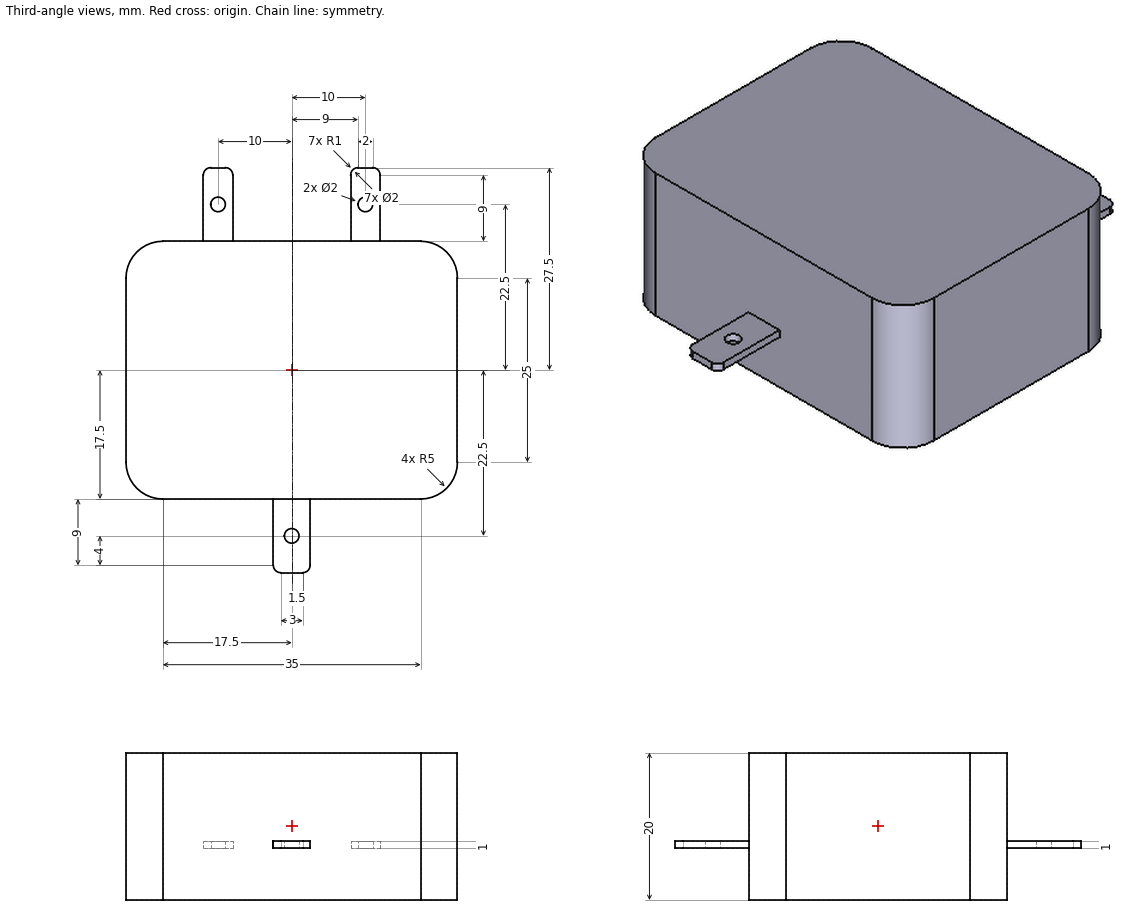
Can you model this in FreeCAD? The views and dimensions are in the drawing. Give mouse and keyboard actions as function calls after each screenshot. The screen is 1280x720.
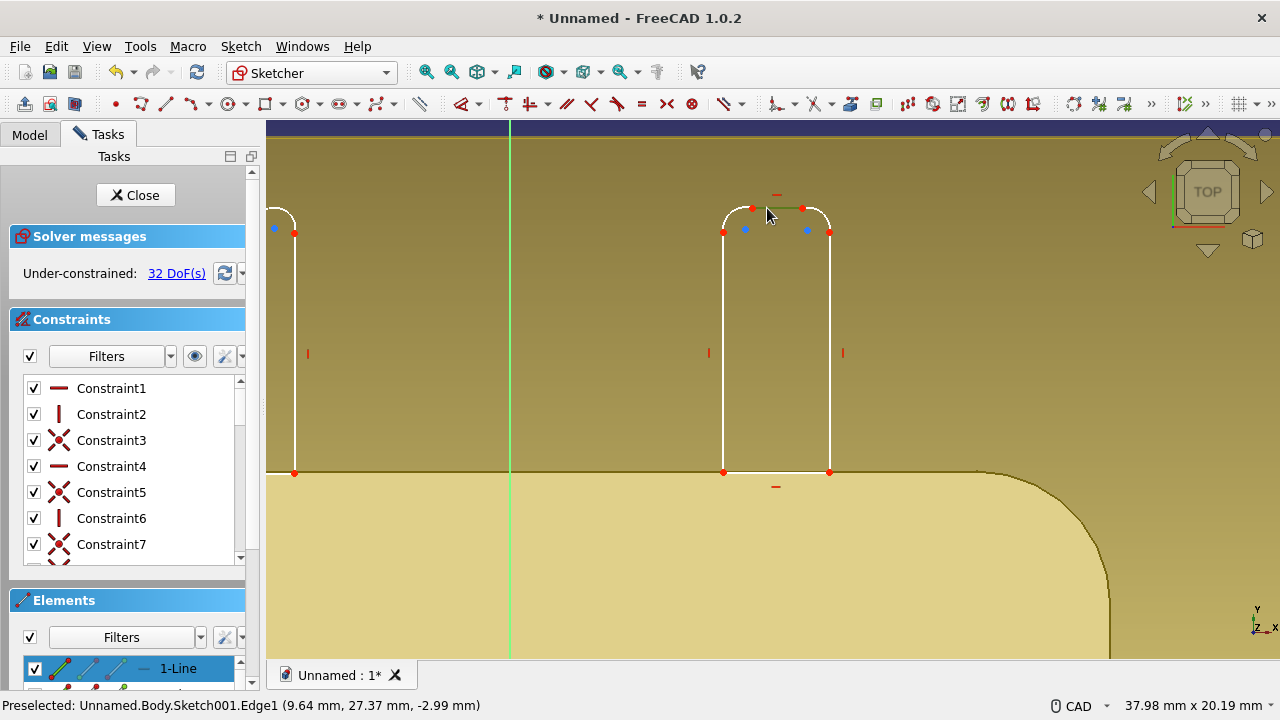
click(828, 220)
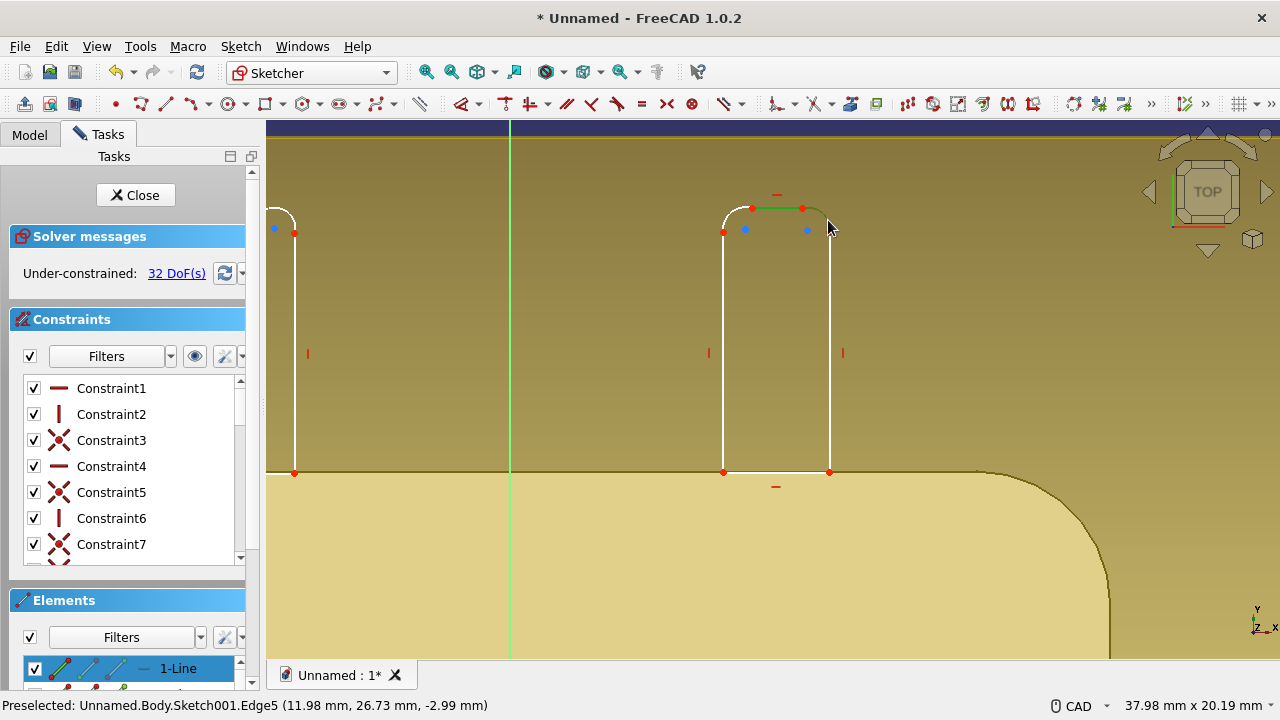
click(617, 104)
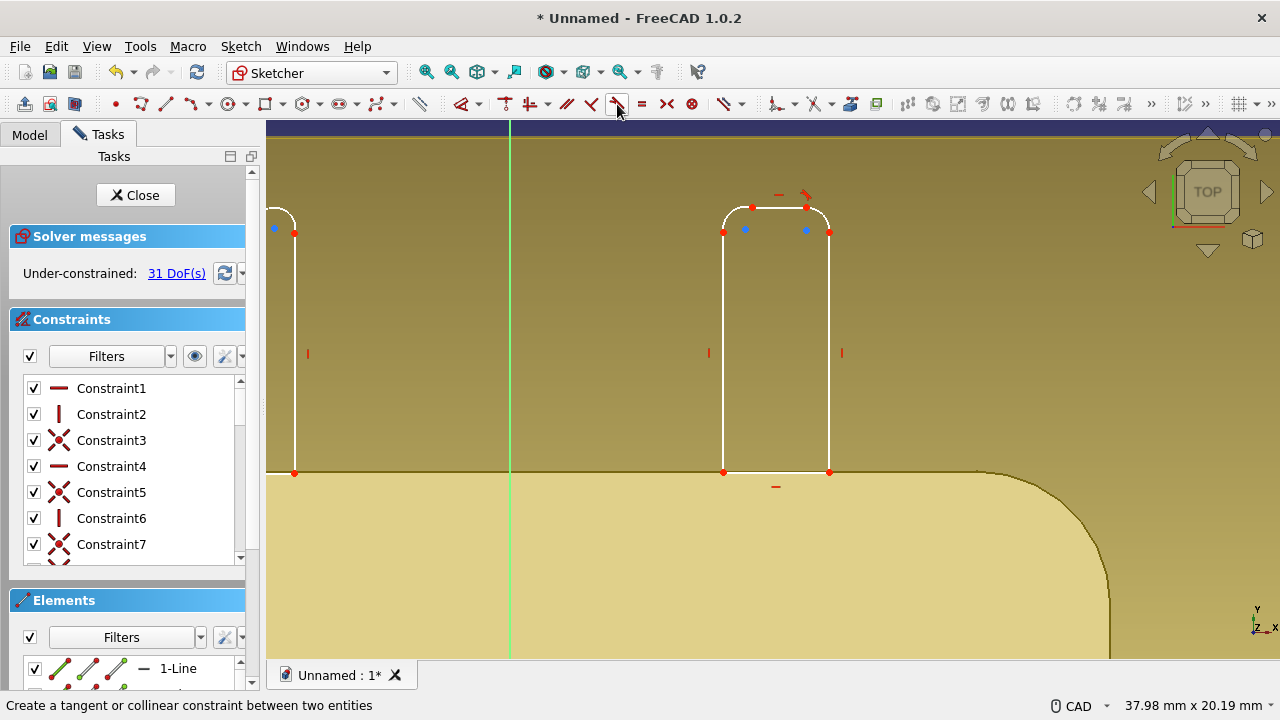
click(769, 208)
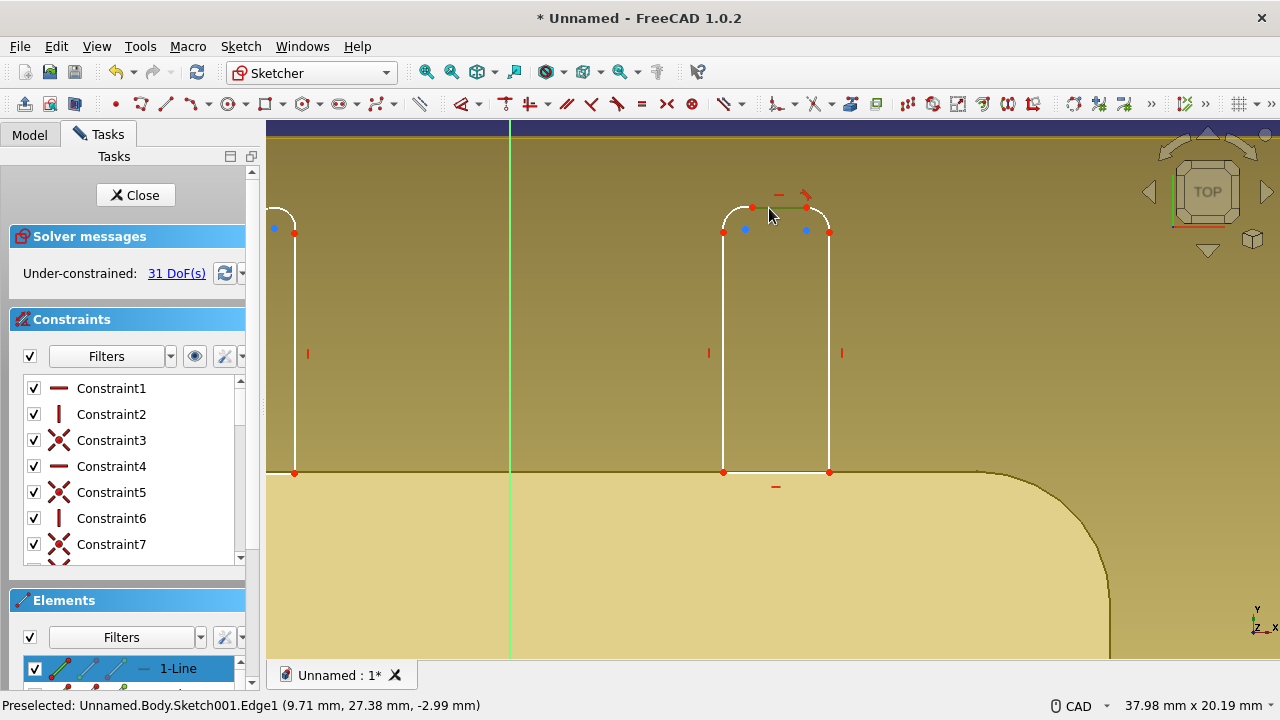
click(739, 208)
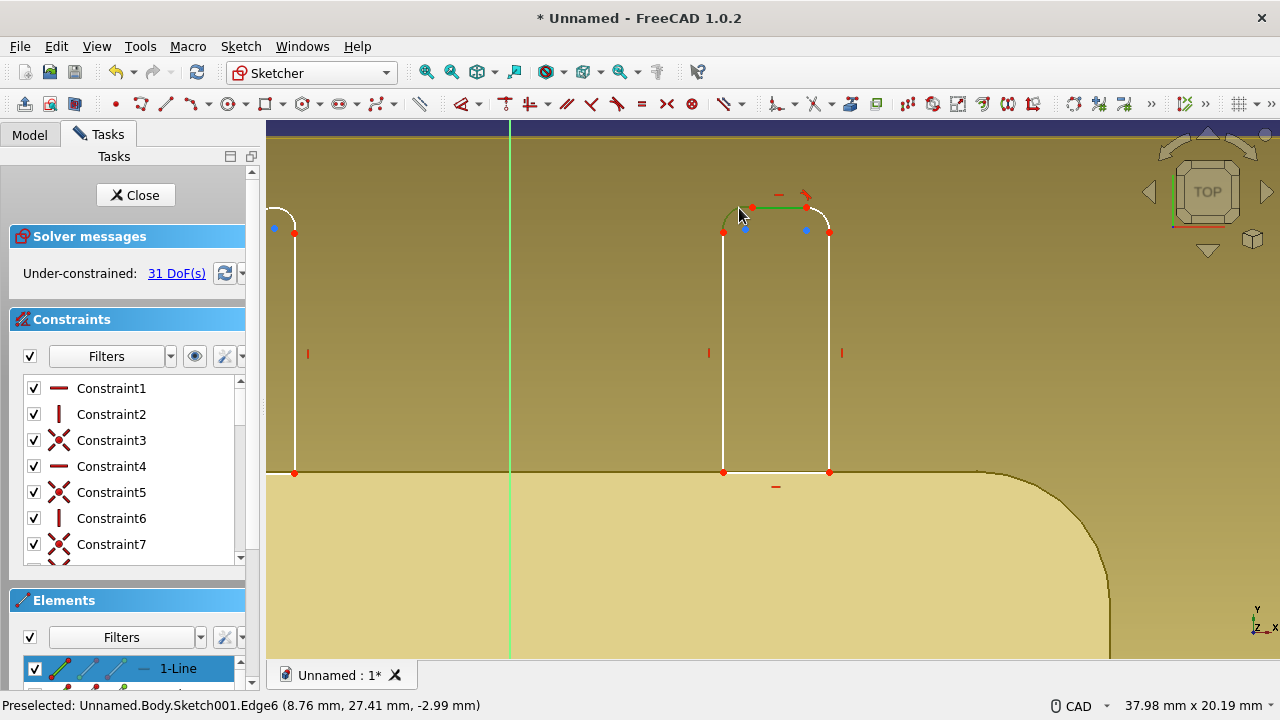
click(617, 104)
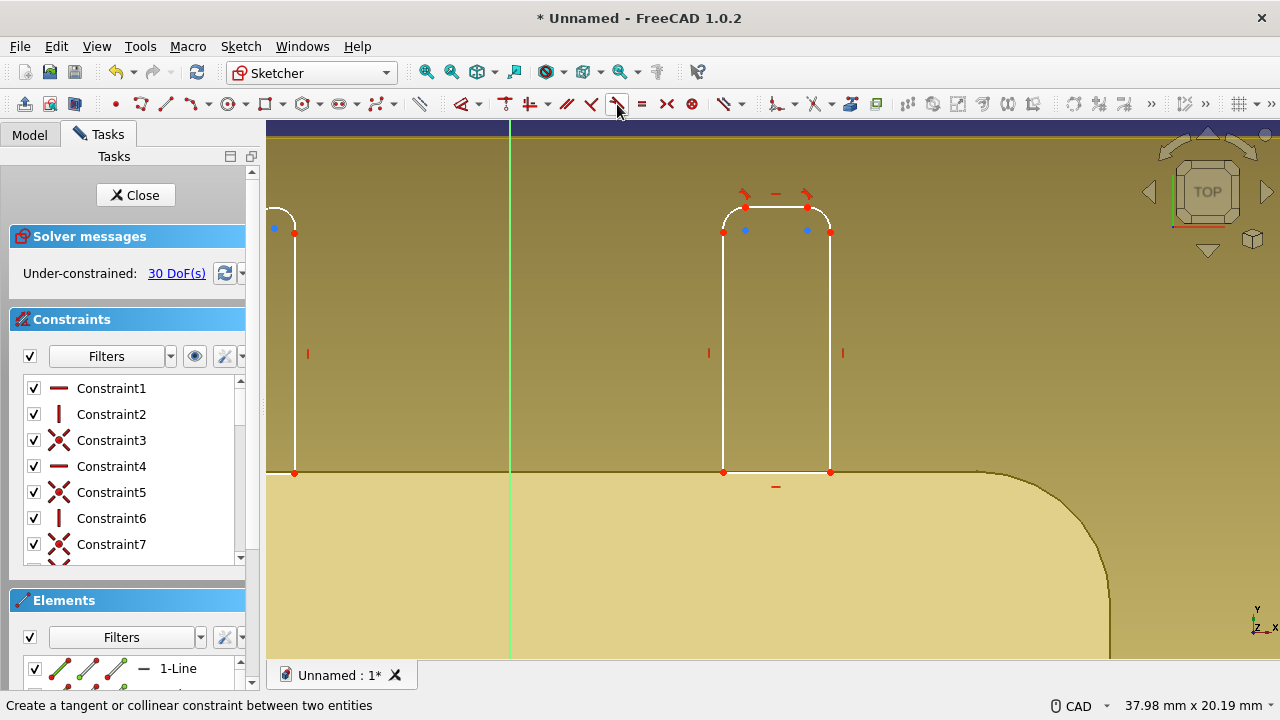
scroll(768, 210, down, 7)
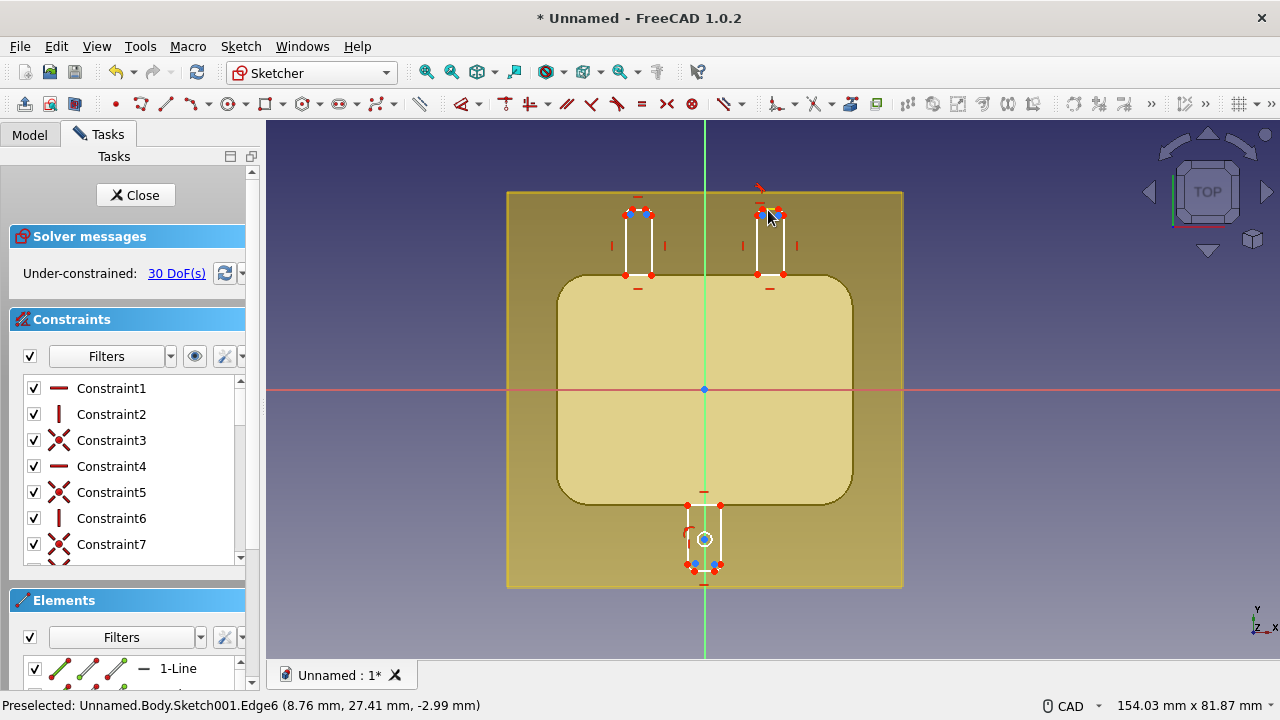
click(784, 234)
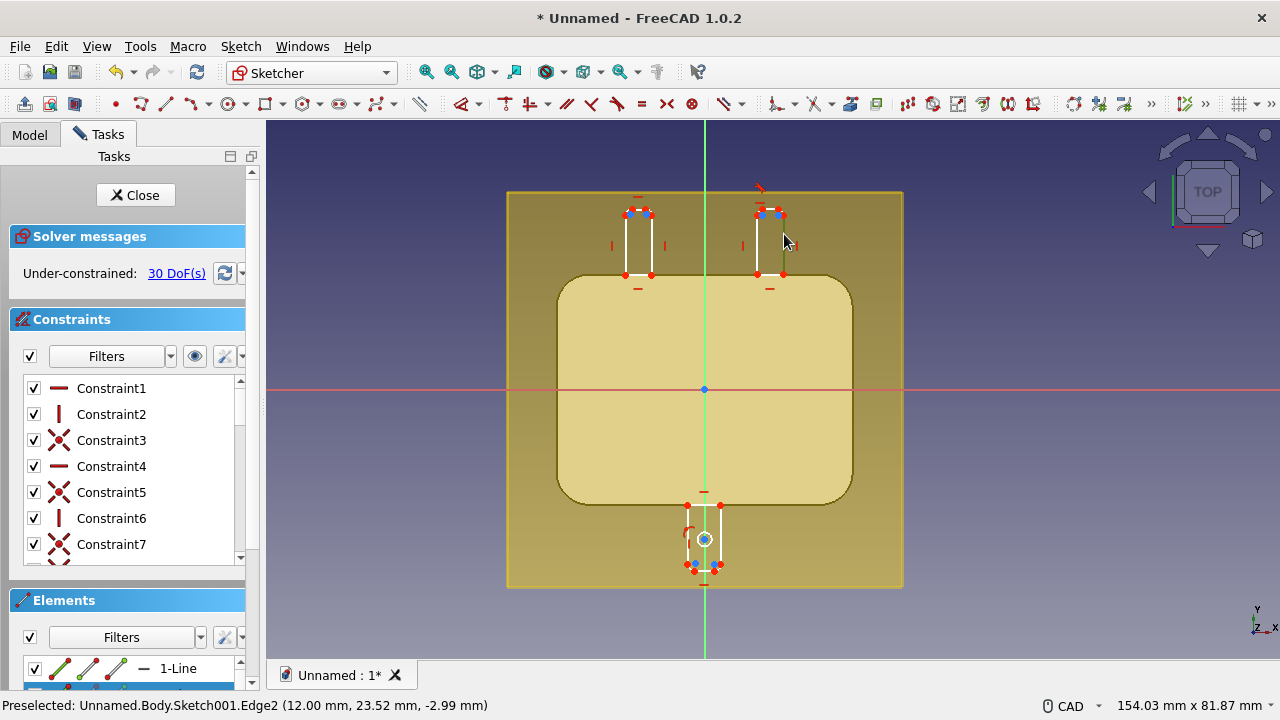
scroll(782, 211, up, 6)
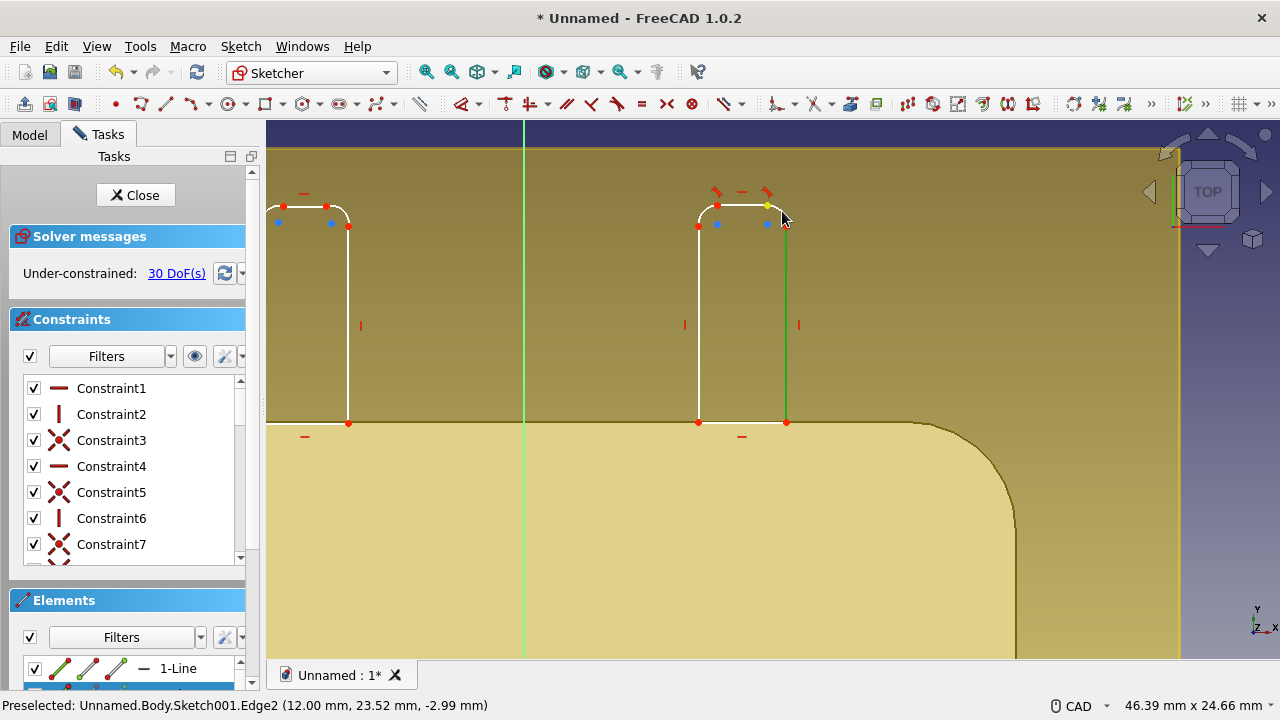
click(782, 212)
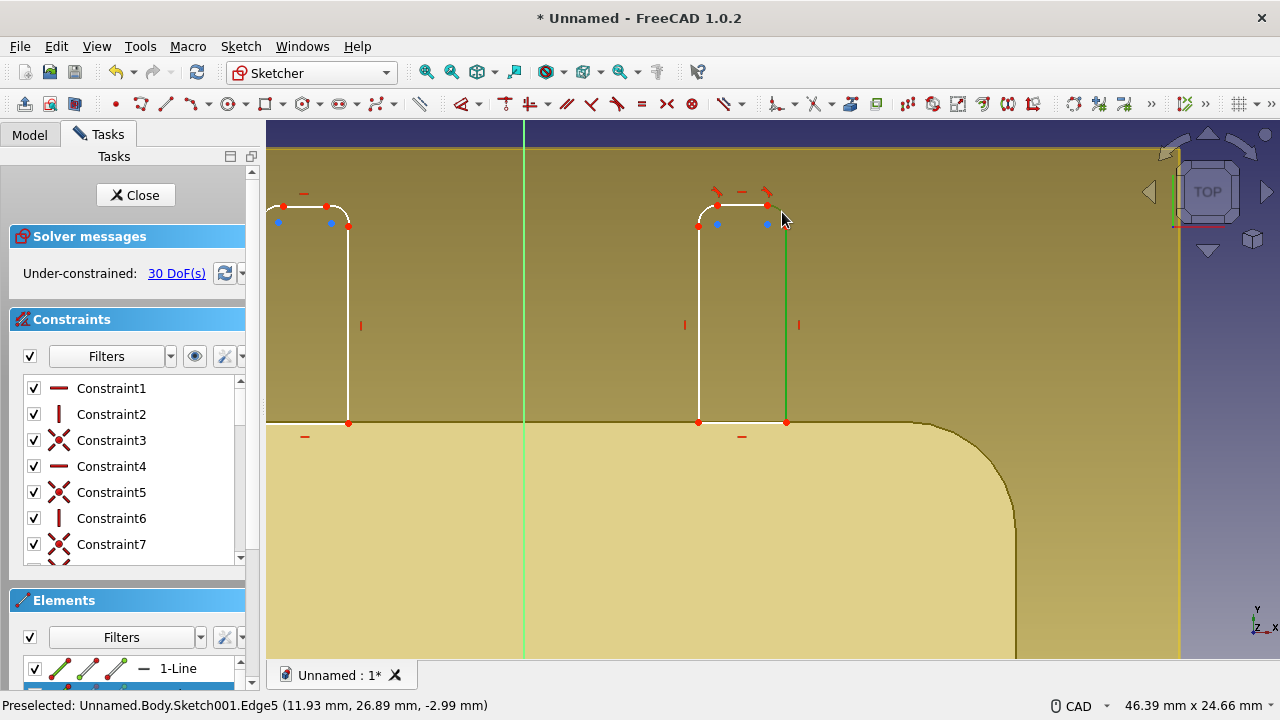
key(t)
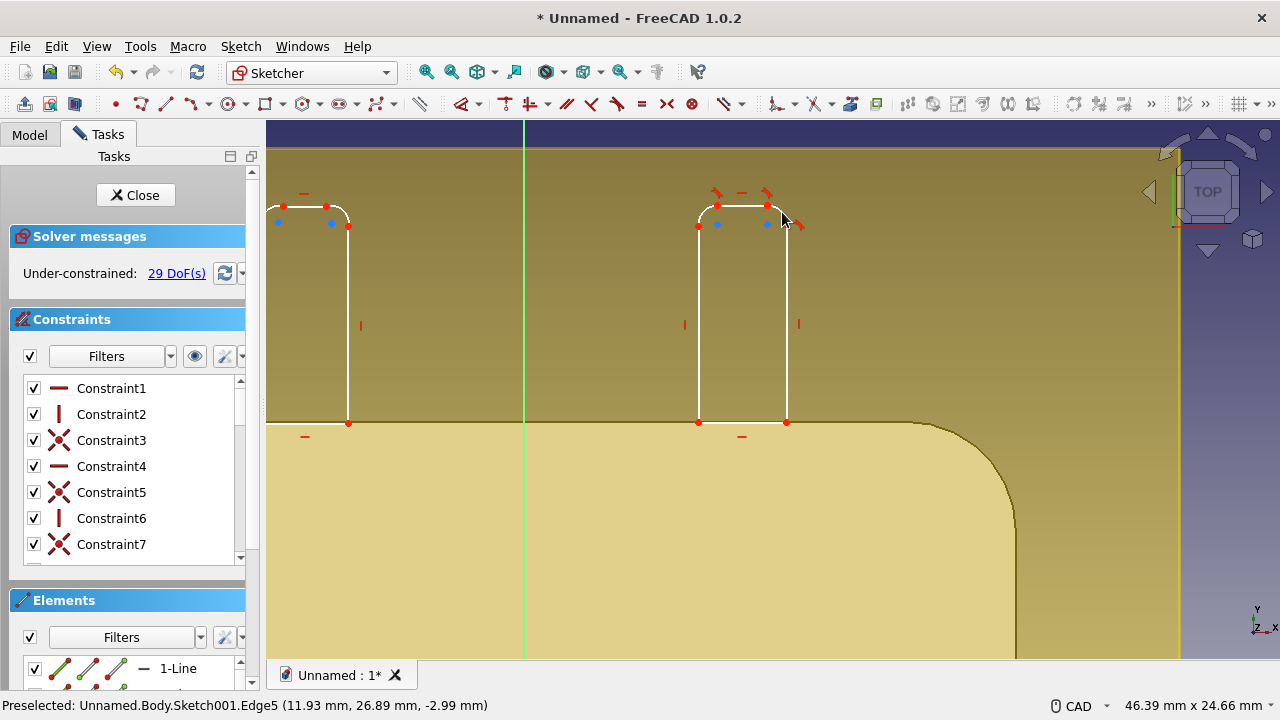
scroll(782, 211, down, 6)